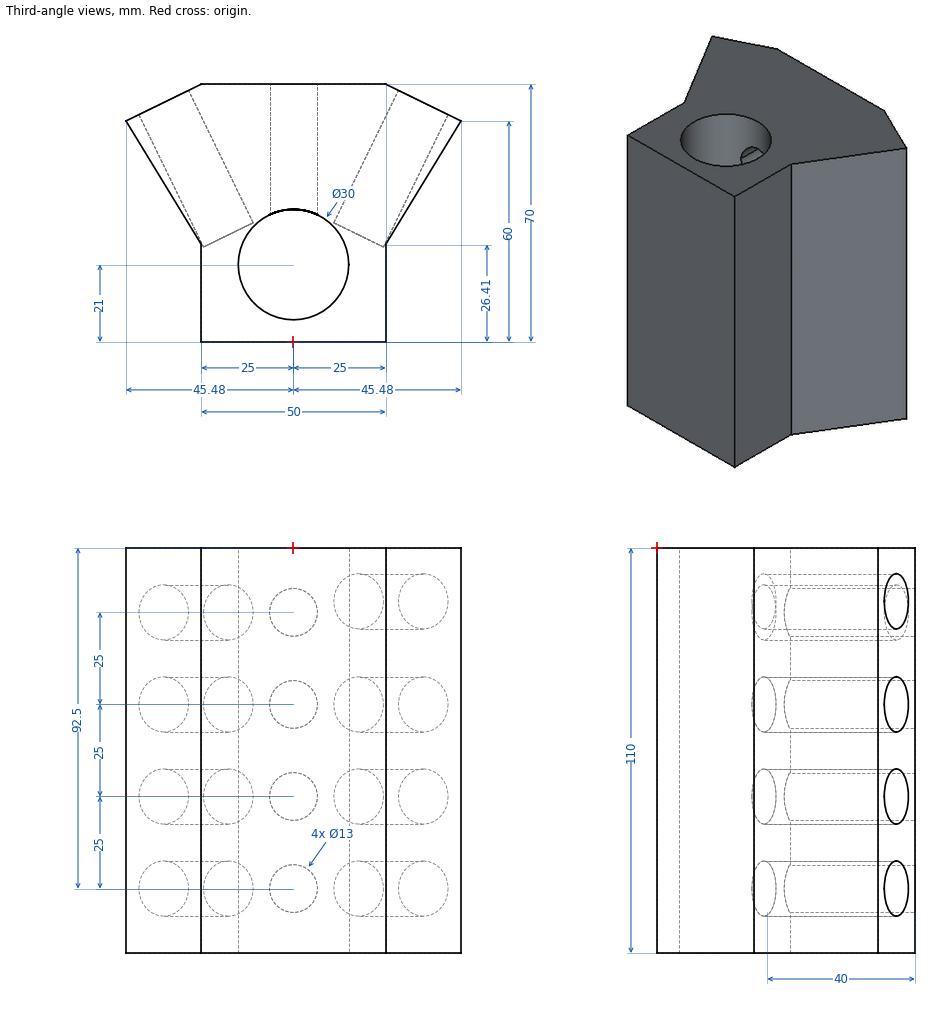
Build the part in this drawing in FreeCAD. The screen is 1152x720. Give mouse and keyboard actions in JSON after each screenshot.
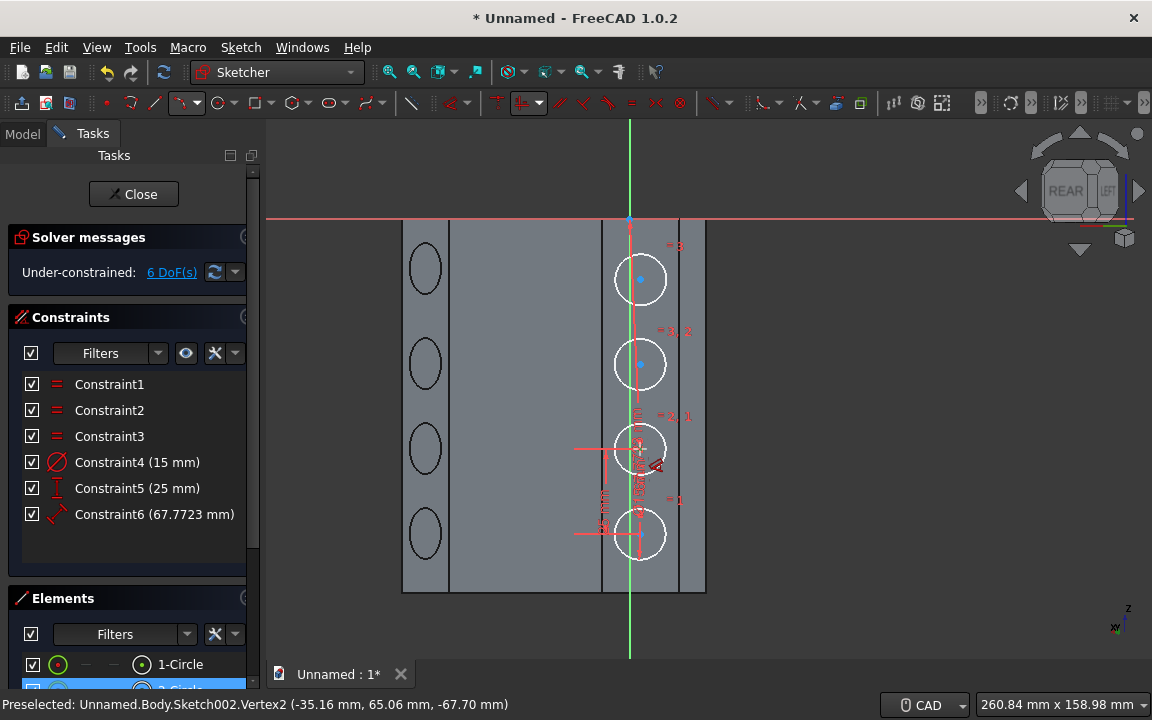
{"action": "left_click", "coordinate": [640, 364]}
{"action": "left_click", "coordinate": [606, 407]}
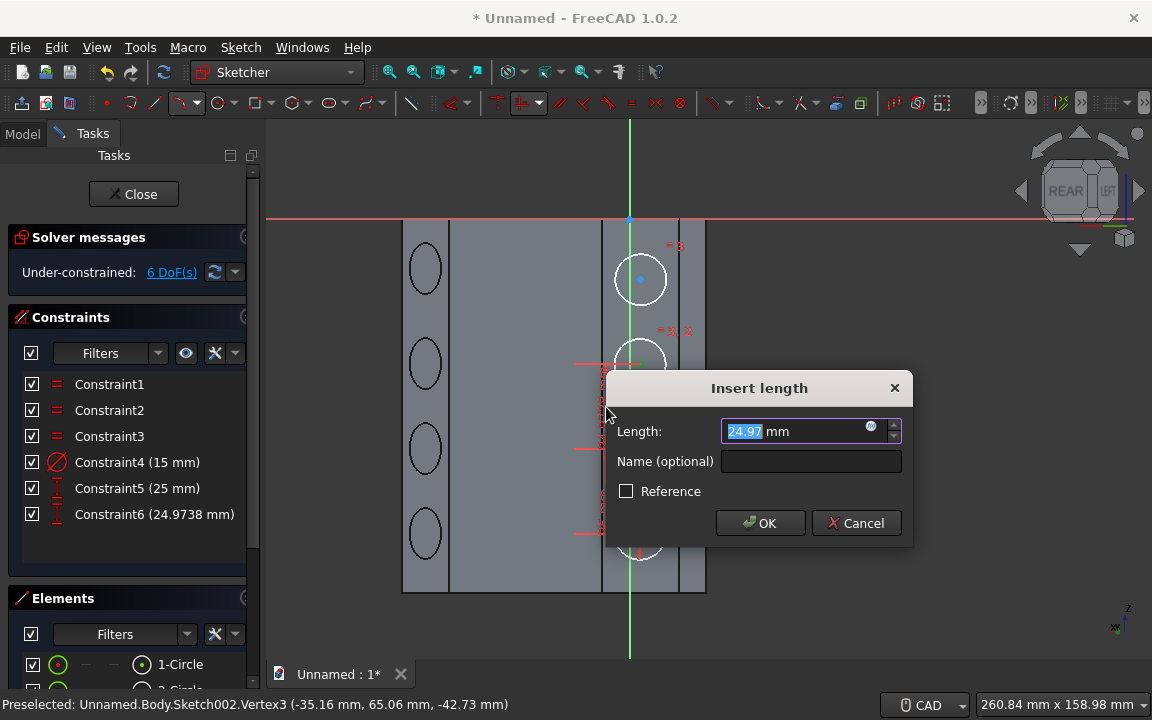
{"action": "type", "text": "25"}
{"action": "key", "text": "Return"}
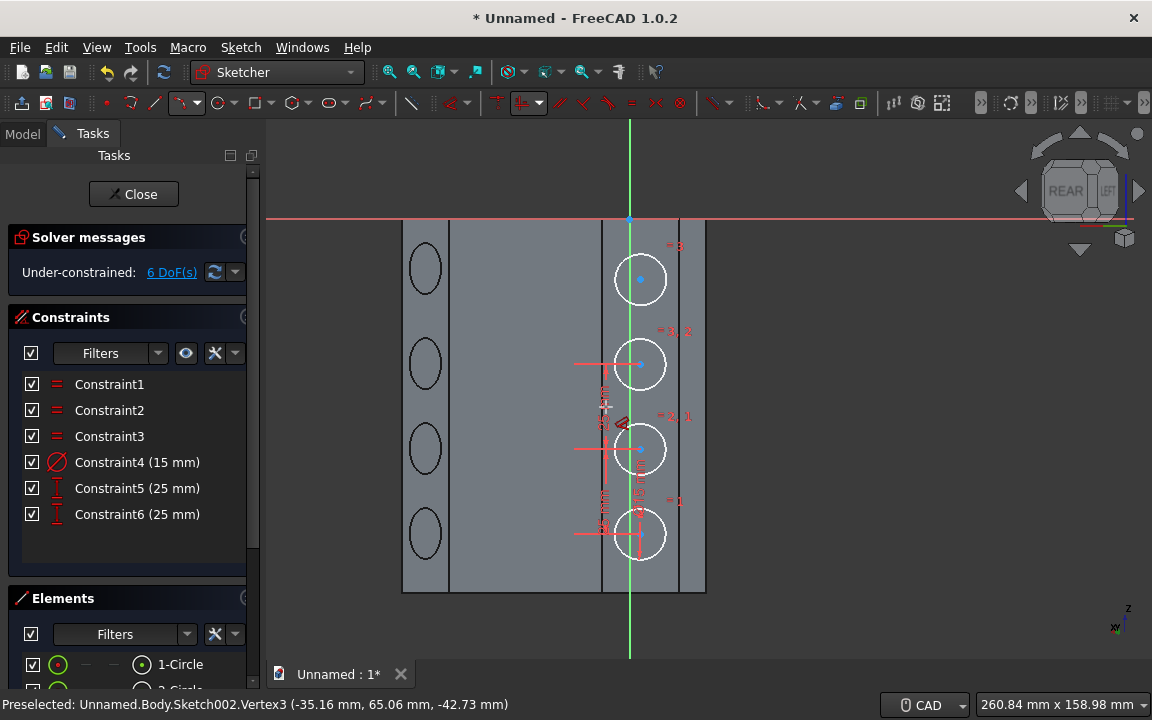
{"action": "left_click", "coordinate": [640, 364]}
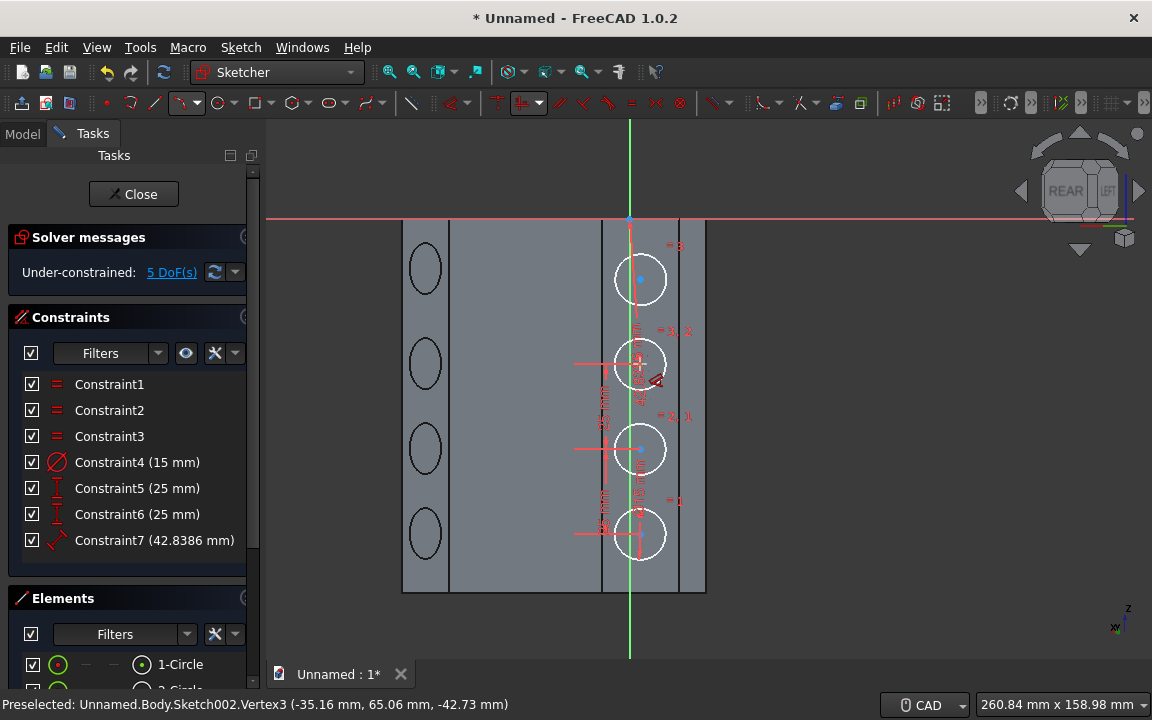
{"action": "left_click", "coordinate": [641, 280]}
{"action": "left_click", "coordinate": [606, 322]}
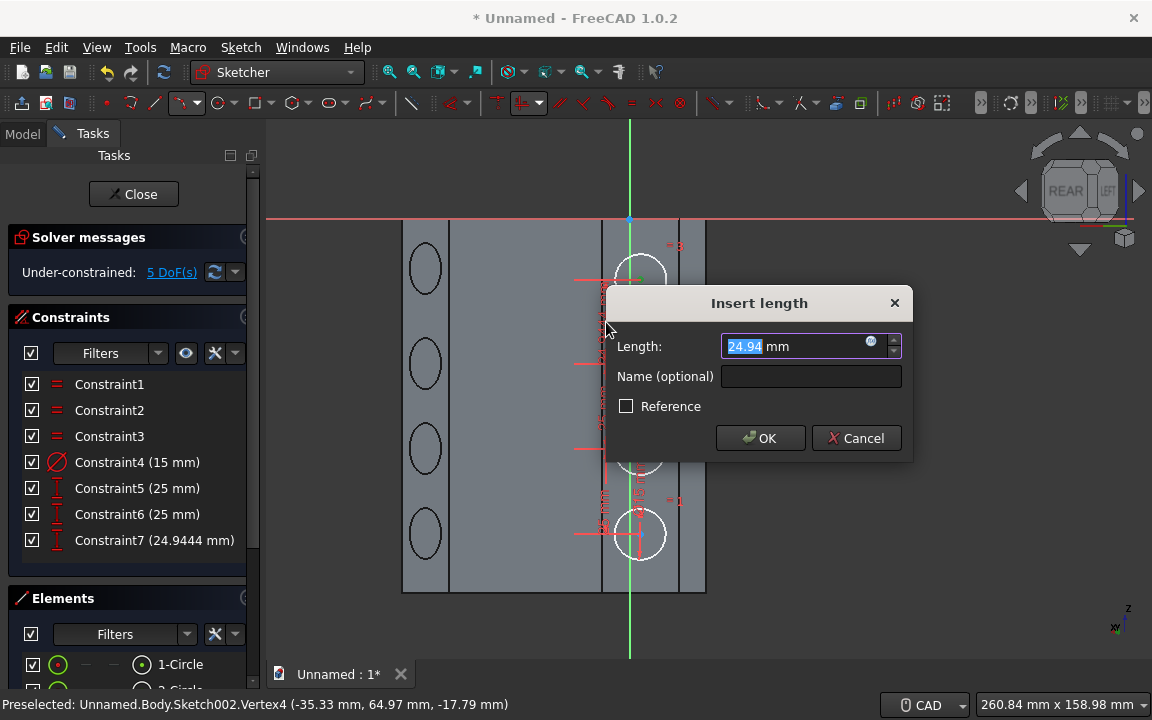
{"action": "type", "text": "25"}
{"action": "key", "text": "Return"}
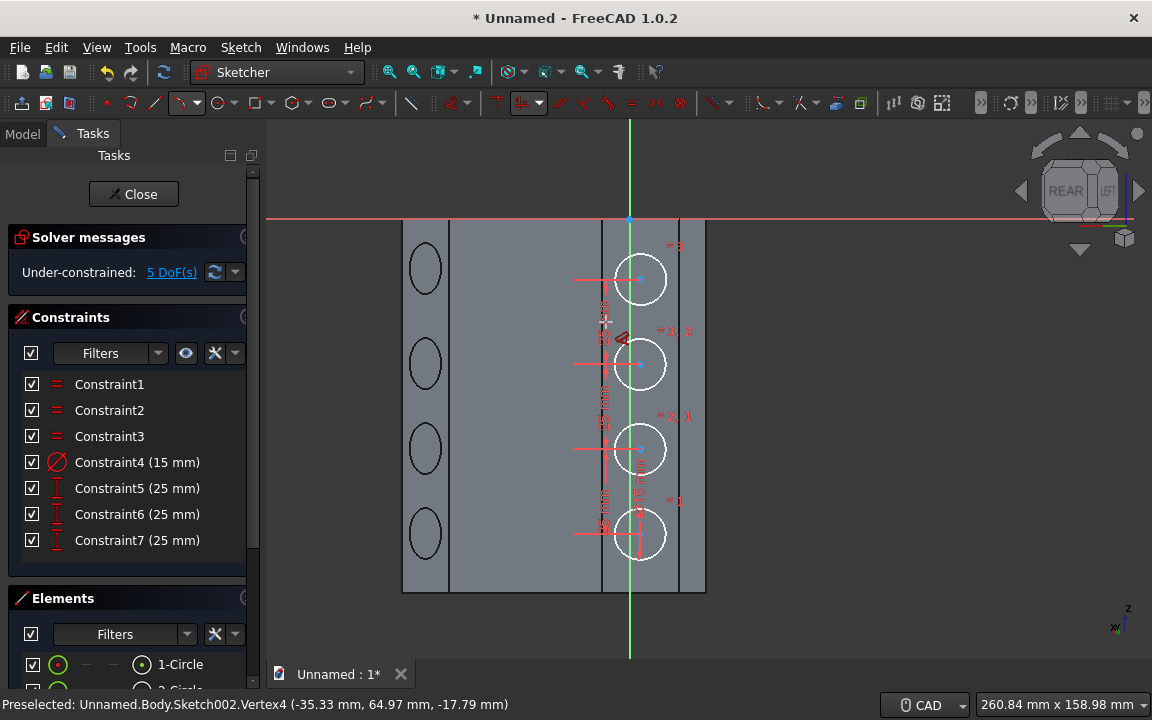
{"action": "left_click", "coordinate": [640, 534]}
{"action": "left_click", "coordinate": [596, 377]}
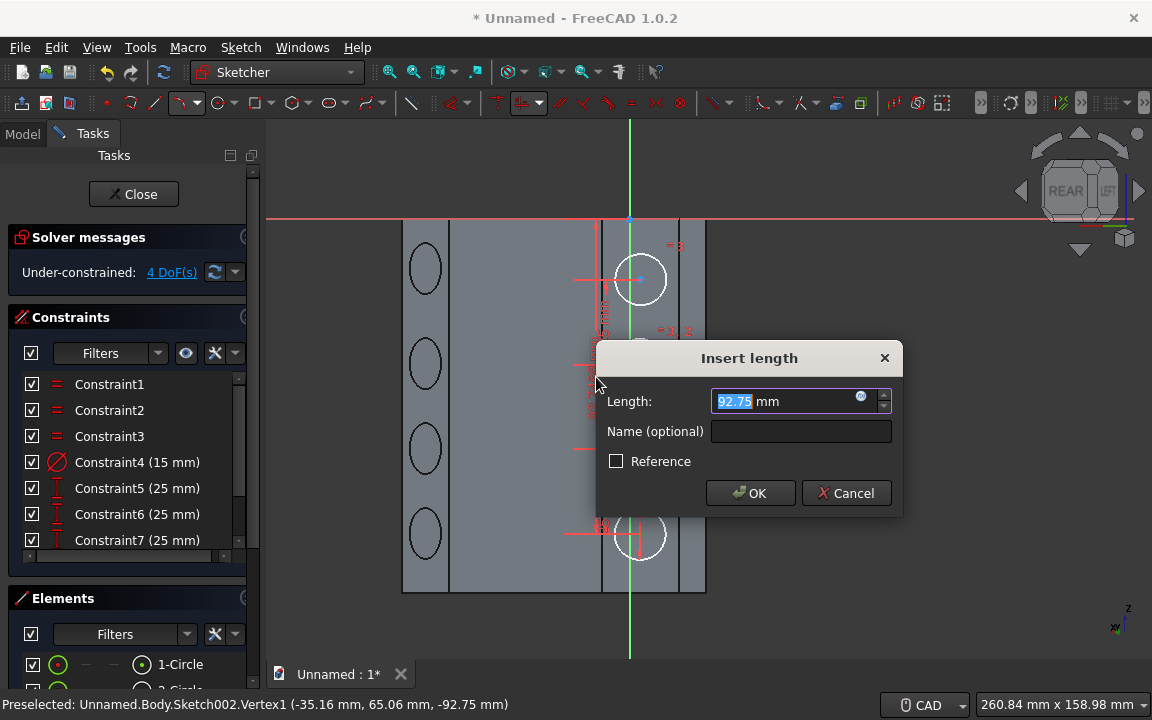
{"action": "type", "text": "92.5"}
{"action": "key", "text": "Return"}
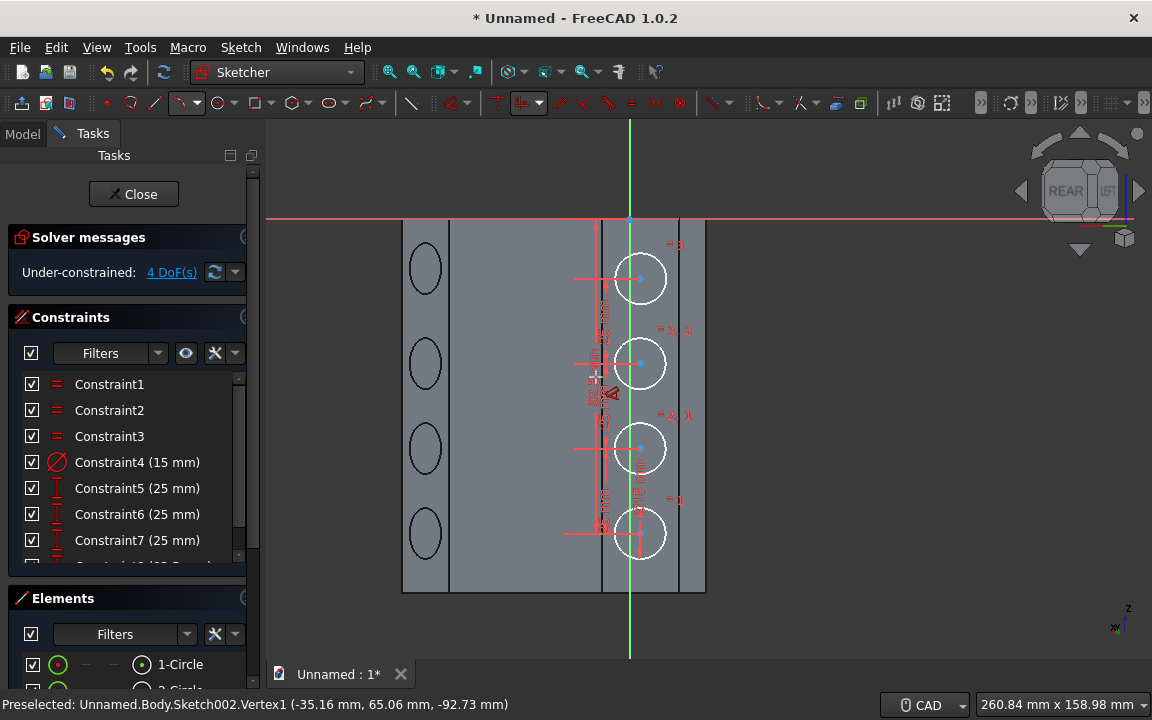
{"action": "scroll", "coordinate": [640, 534], "scroll_direction": "up", "scroll_amount": 7}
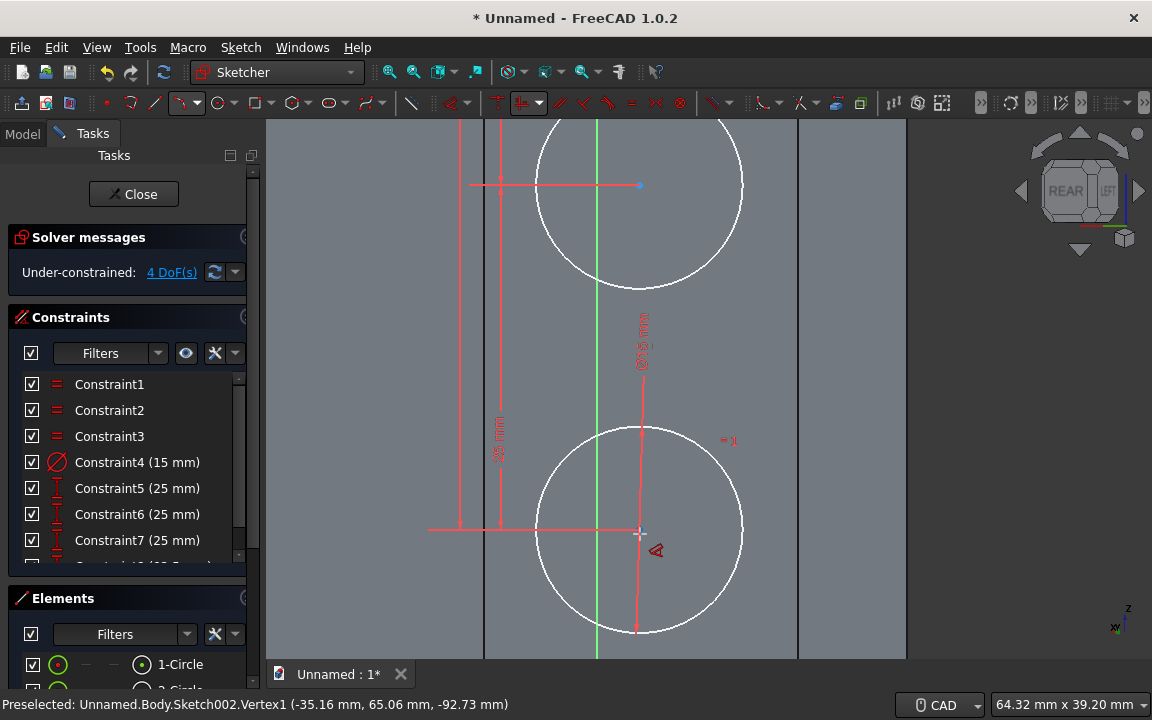
{"action": "left_click", "coordinate": [639, 530]}
{"action": "left_click", "coordinate": [618, 564]}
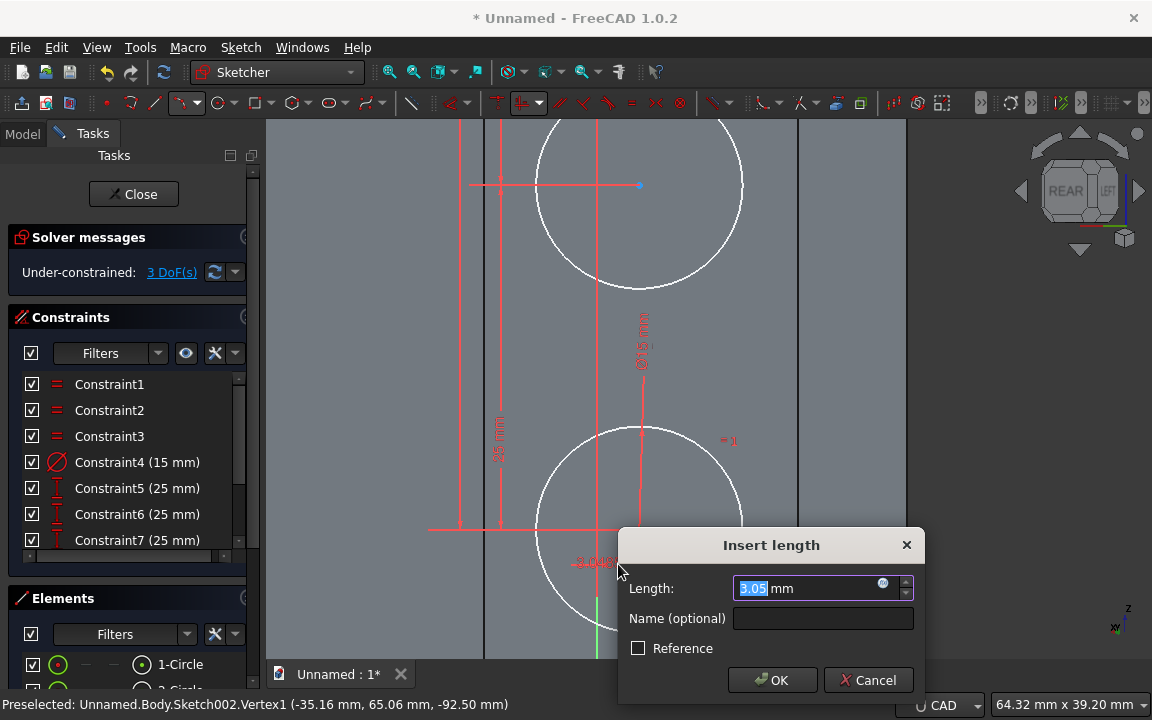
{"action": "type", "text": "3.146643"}
{"action": "key", "text": "Return"}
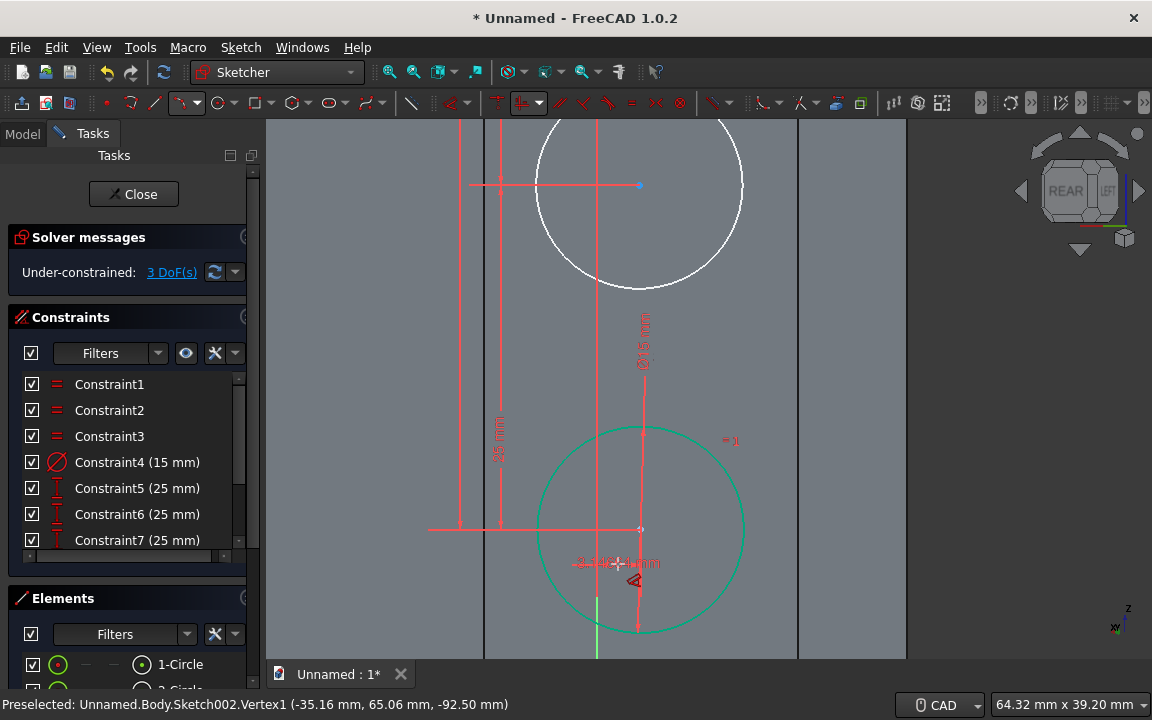
{"action": "left_click", "coordinate": [639, 185]}
{"action": "left_click", "coordinate": [618, 219]}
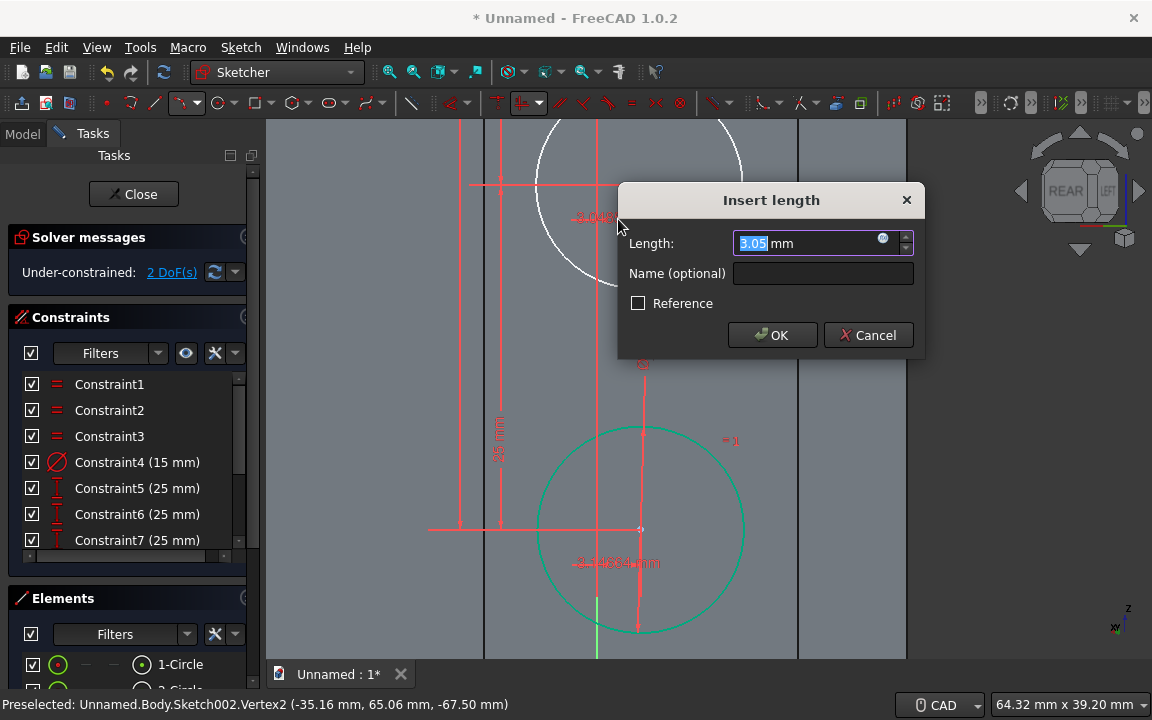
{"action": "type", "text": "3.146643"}
{"action": "key", "text": "Return"}